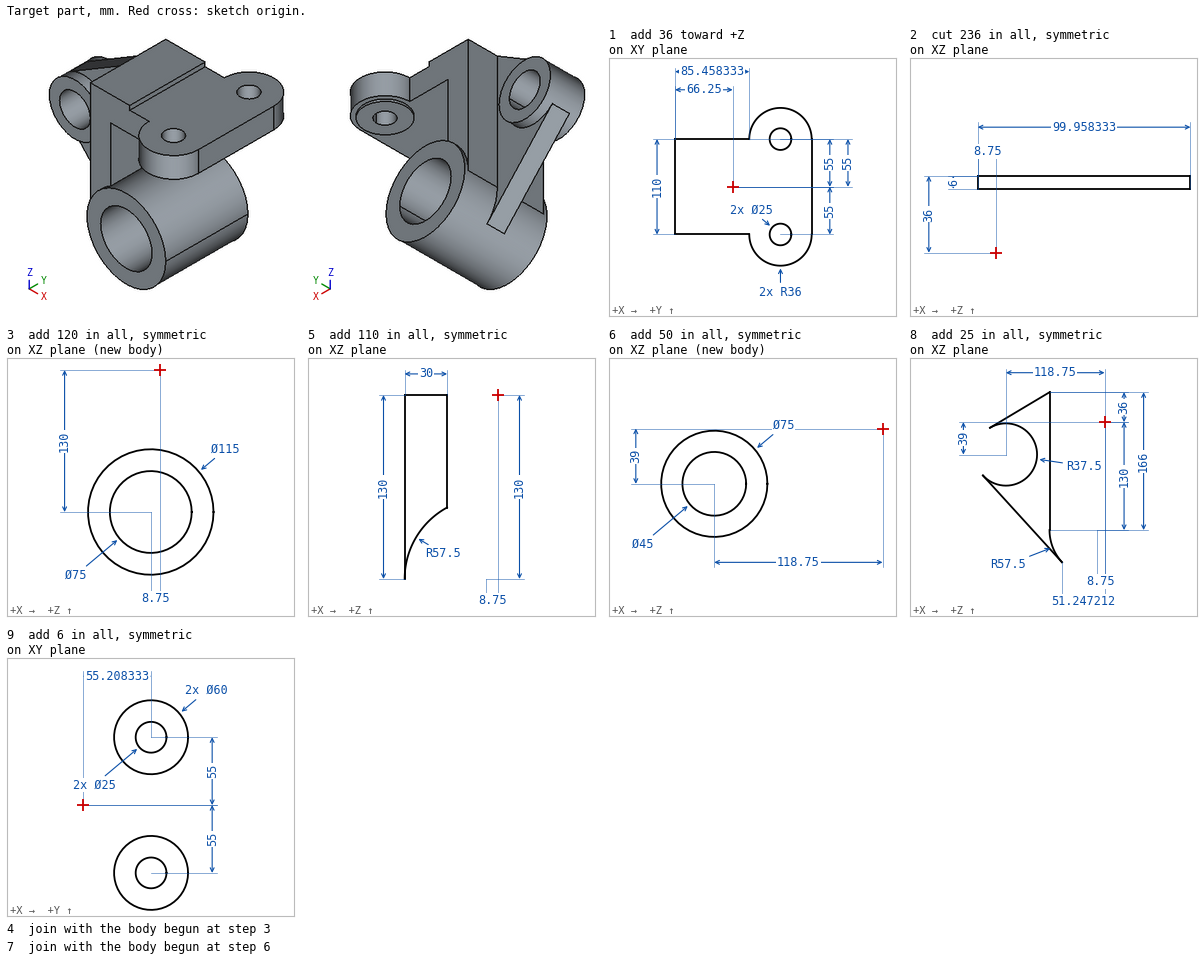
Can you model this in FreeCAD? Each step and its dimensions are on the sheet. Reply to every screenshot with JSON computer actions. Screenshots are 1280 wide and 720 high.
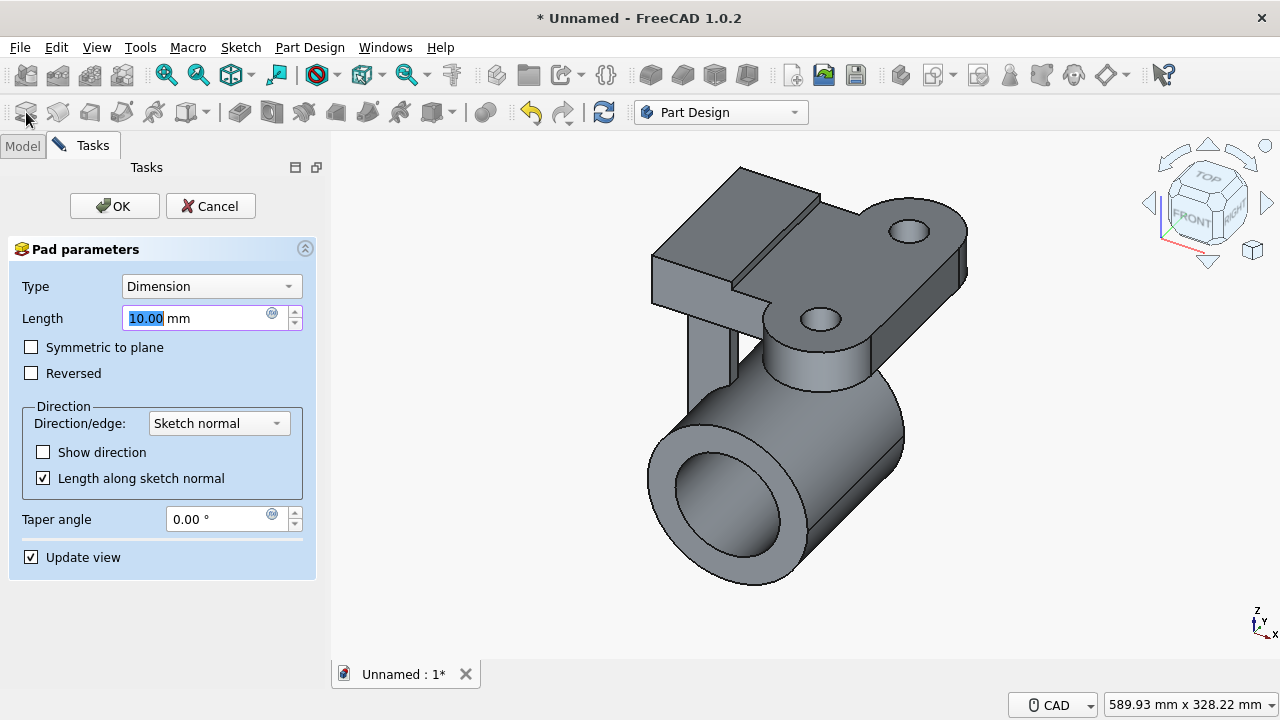
{"action": "type", "text": "110"}
{"action": "key", "text": "Tab"}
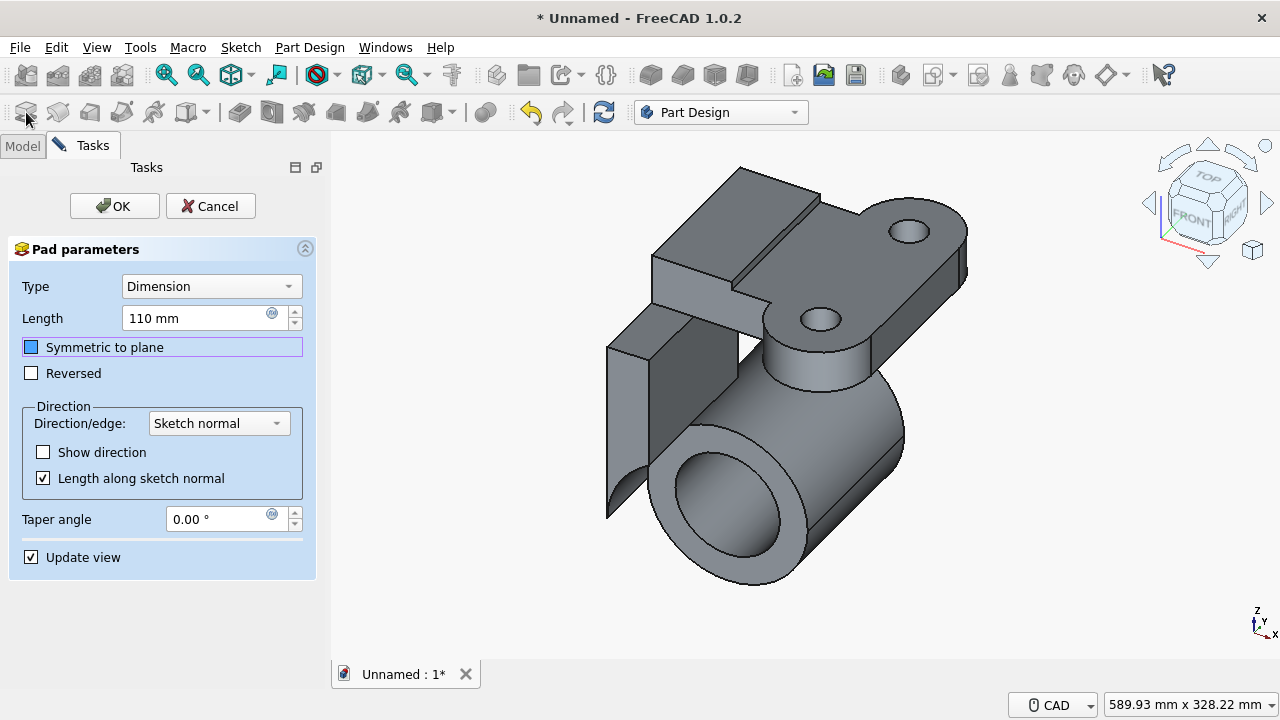
{"action": "left_click", "coordinate": [30, 347]}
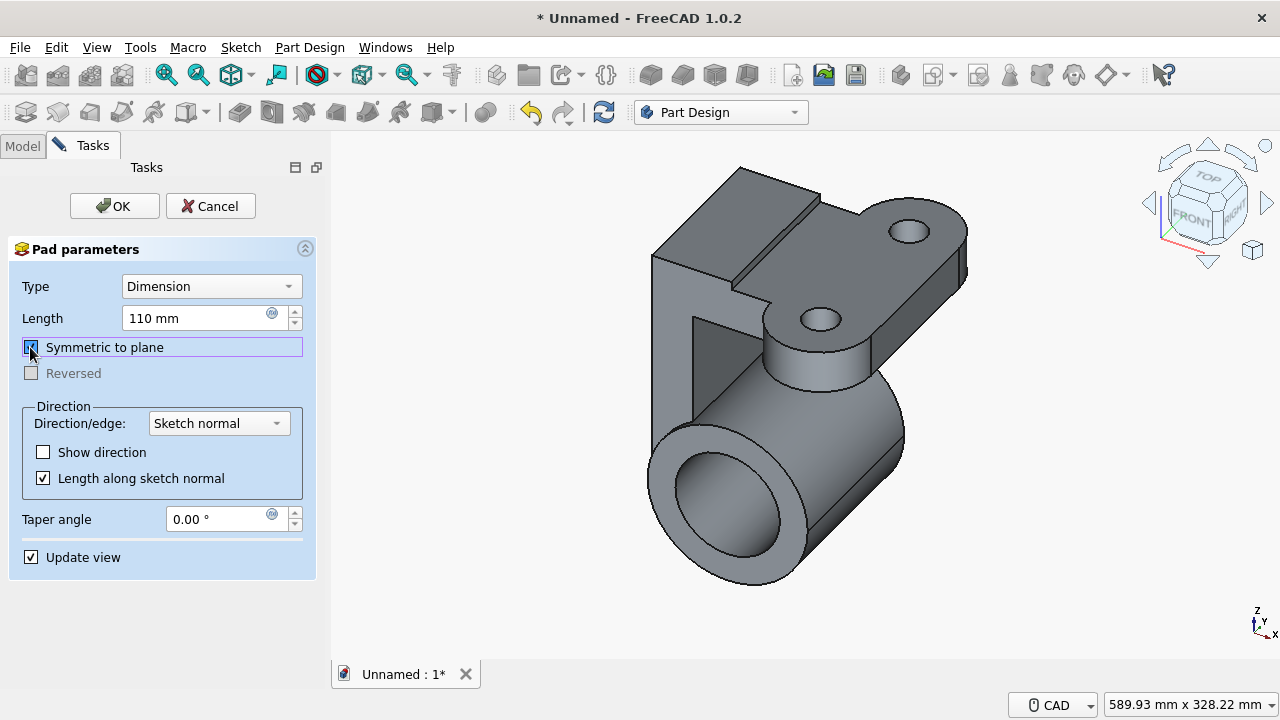
{"action": "left_click", "coordinate": [115, 206]}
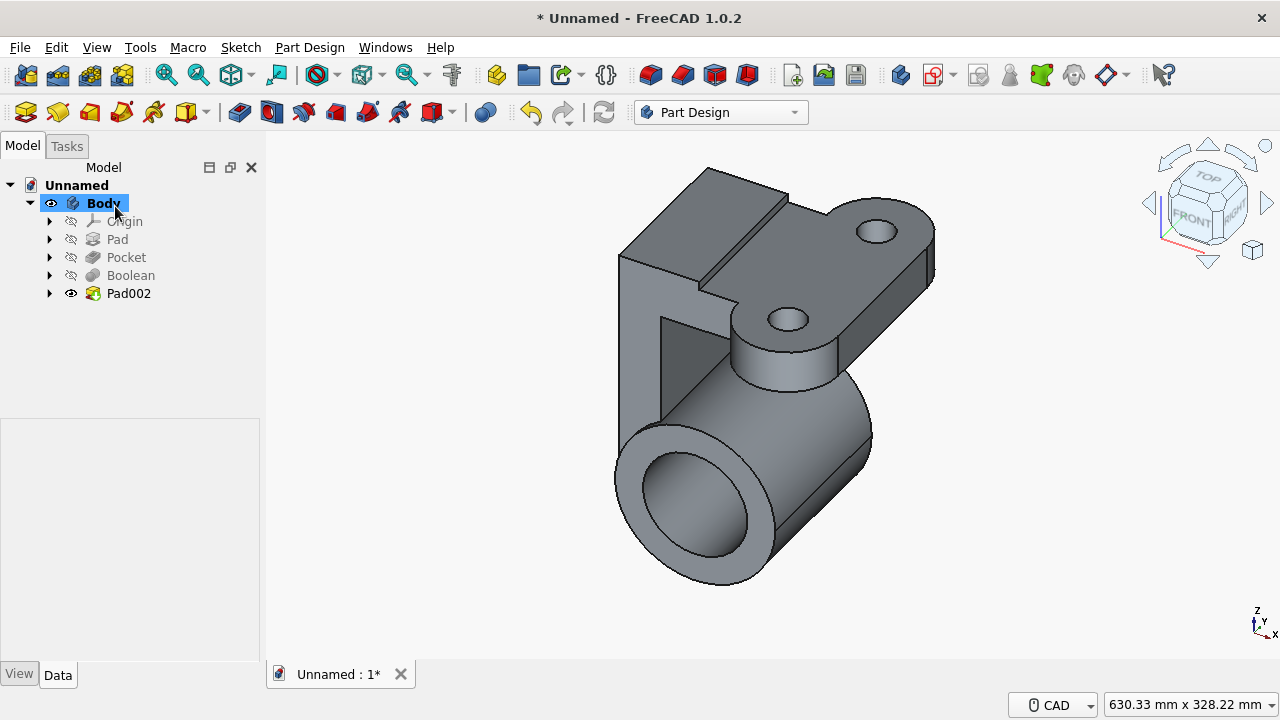
{"action": "left_click", "coordinate": [902, 76]}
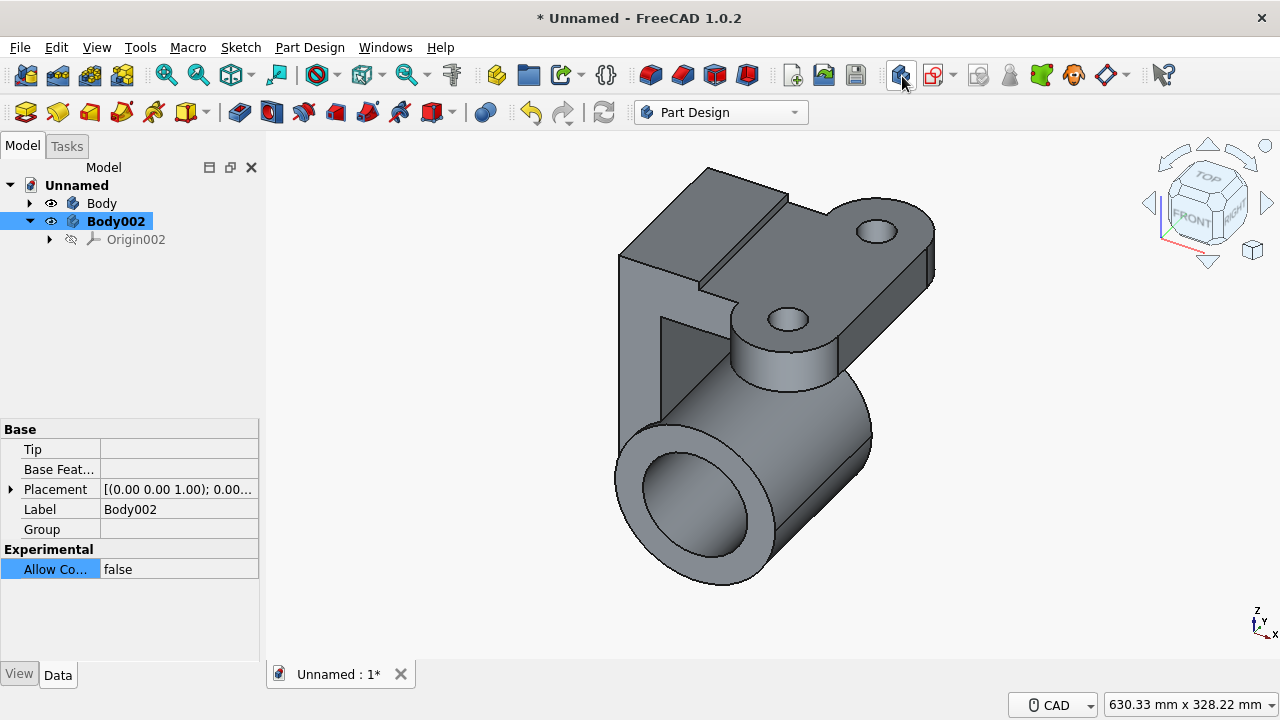
{"action": "left_click", "coordinate": [306, 619]}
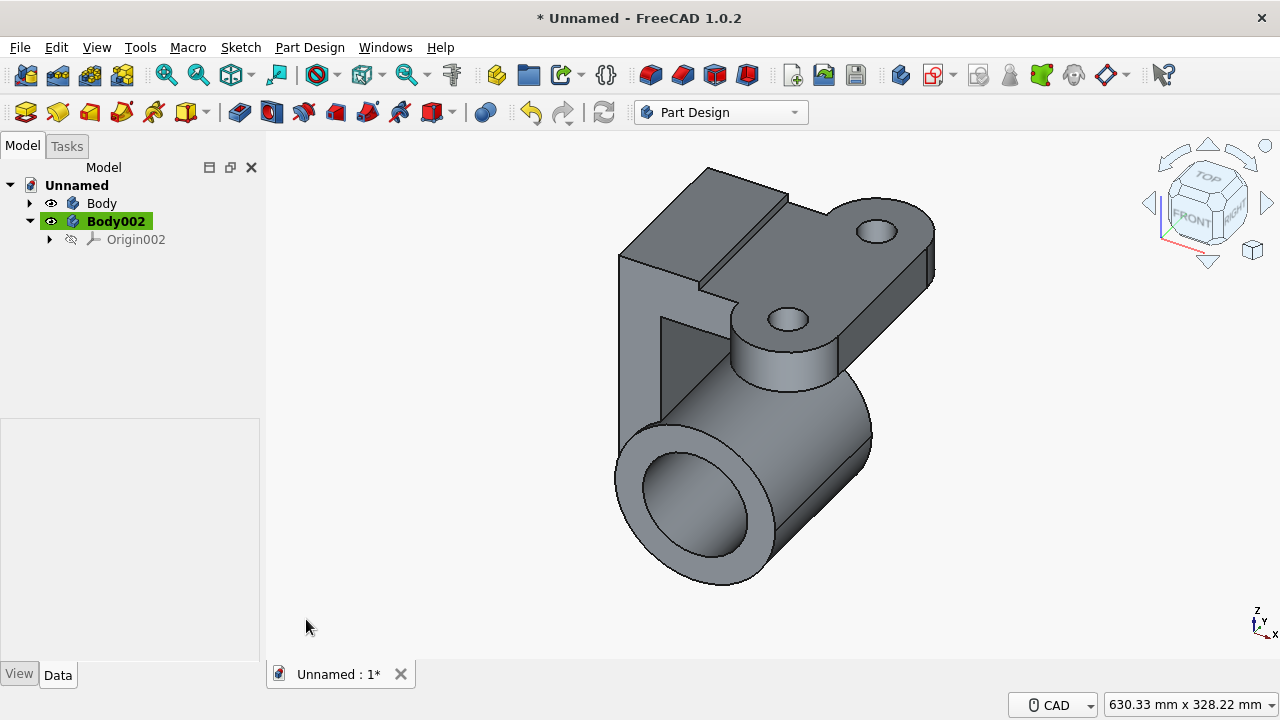
{"action": "left_click", "coordinate": [934, 76]}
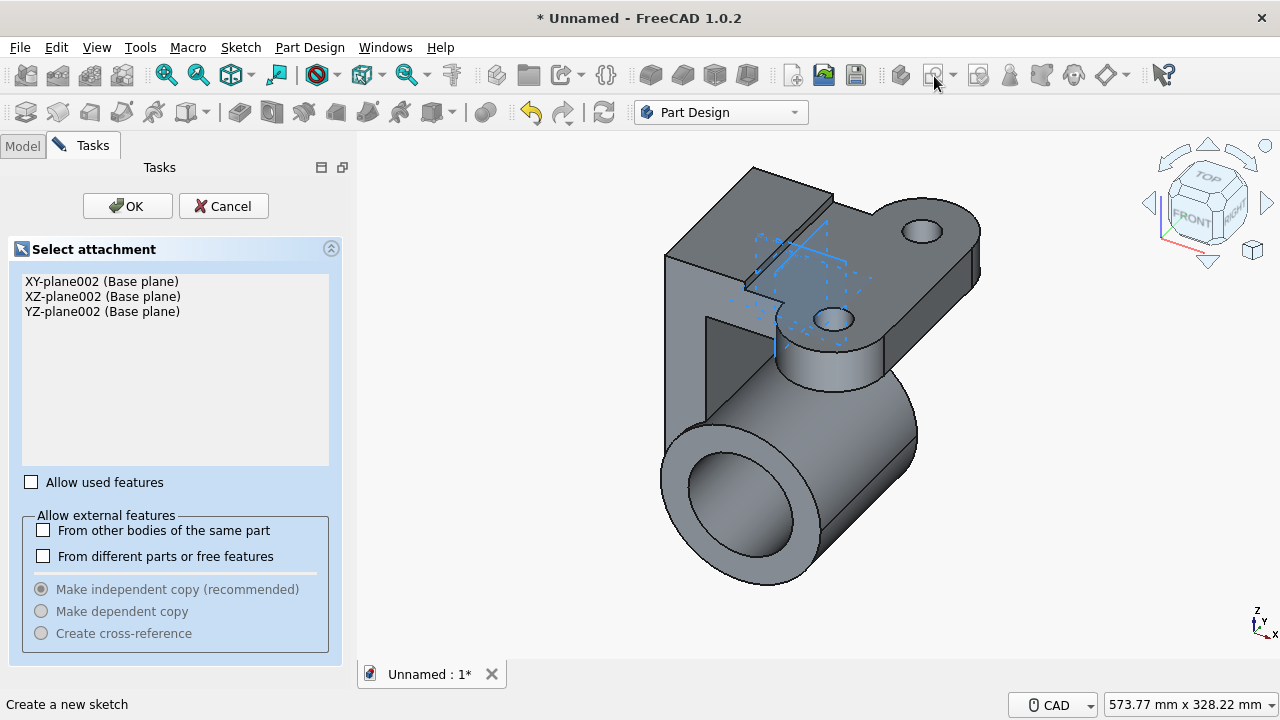
{"action": "left_click", "coordinate": [82, 296]}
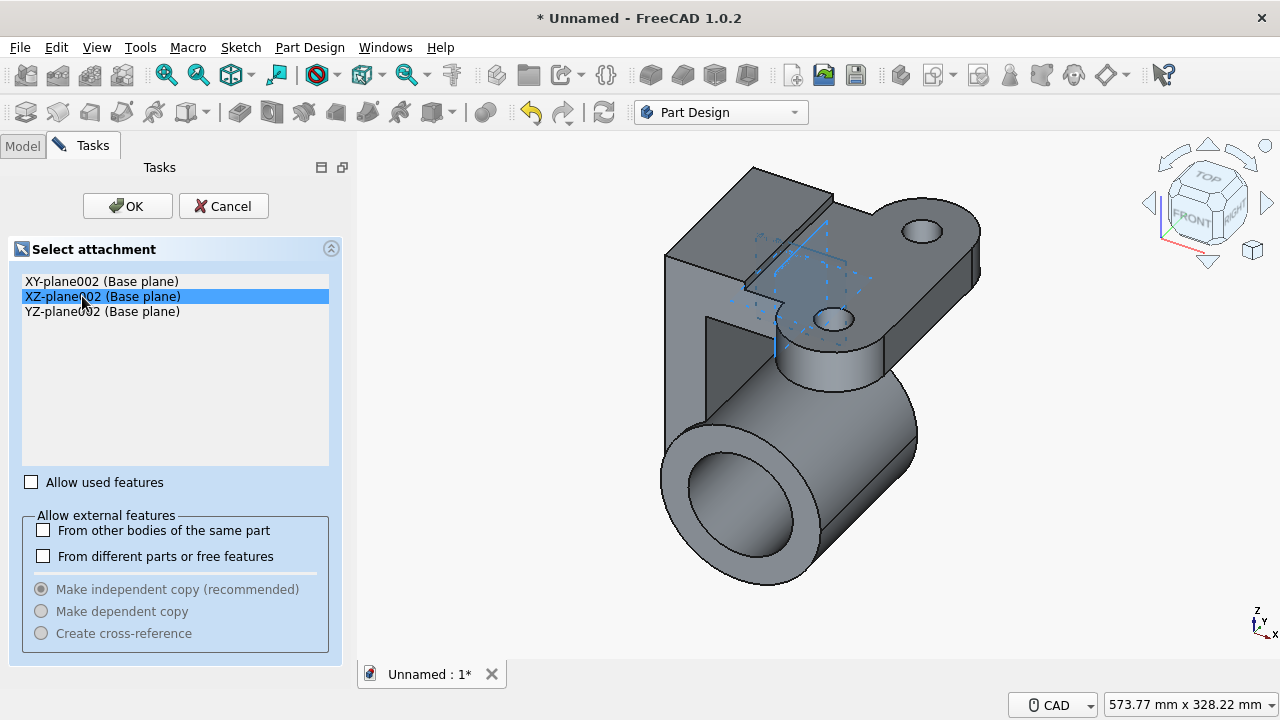
{"action": "left_click", "coordinate": [128, 206]}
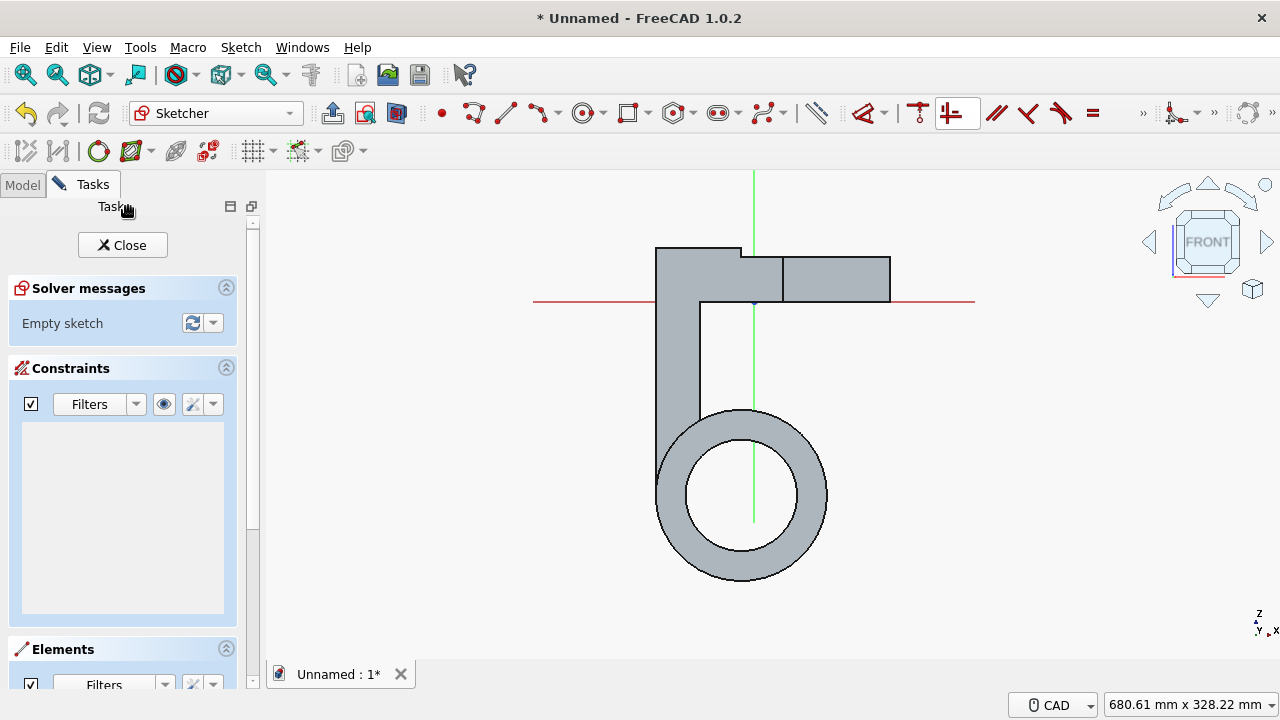
{"action": "scroll", "coordinate": [599, 326], "scroll_direction": "up", "scroll_amount": 5}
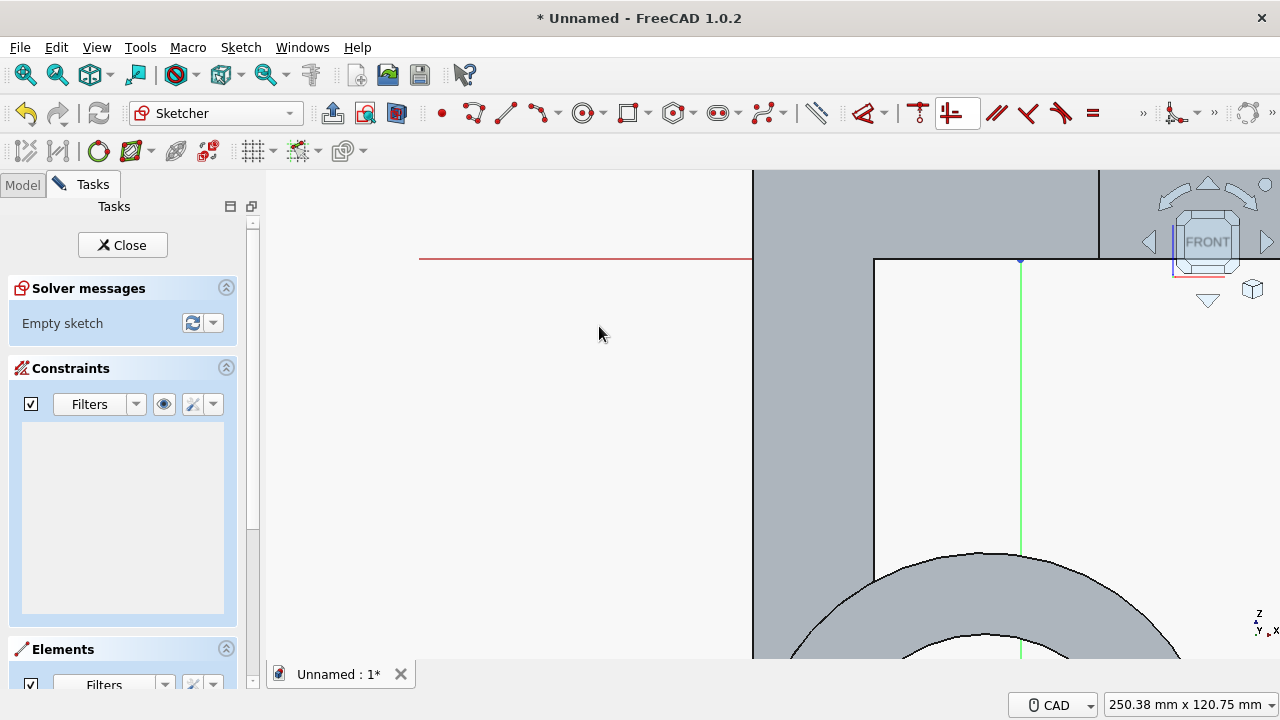
{"action": "left_click", "coordinate": [584, 114]}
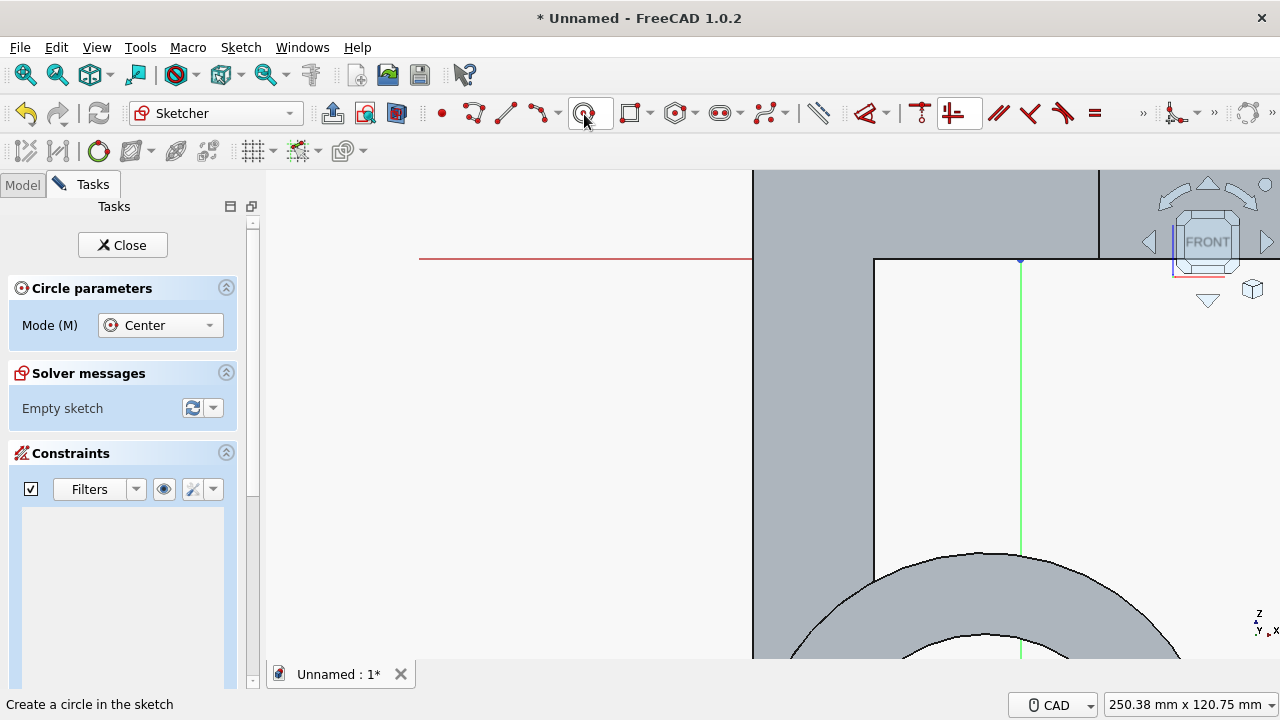
{"action": "left_click", "coordinate": [540, 417]}
{"action": "left_click", "coordinate": [647, 310]}